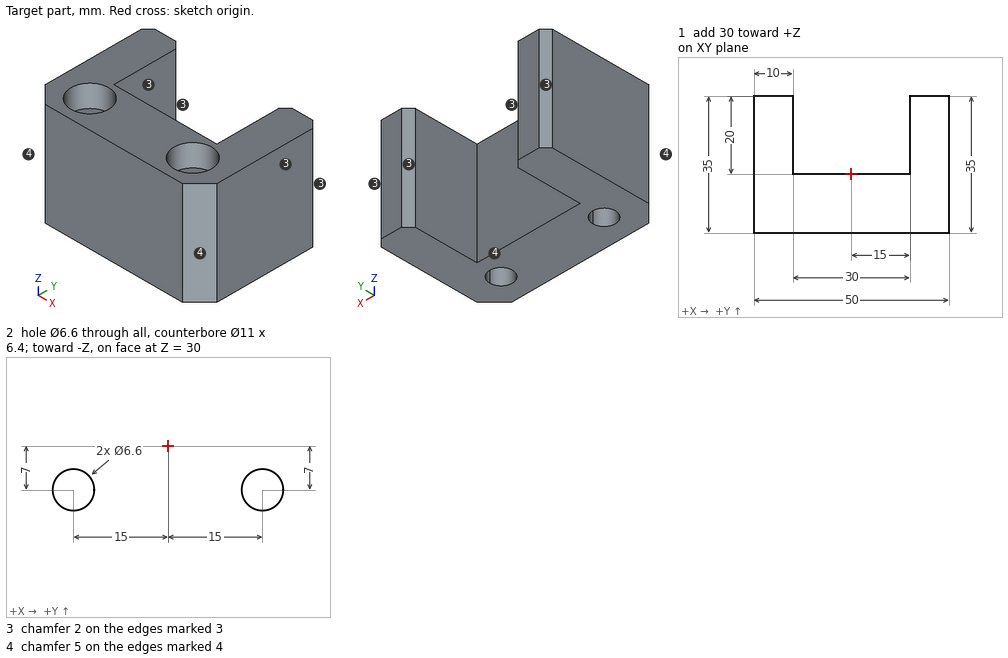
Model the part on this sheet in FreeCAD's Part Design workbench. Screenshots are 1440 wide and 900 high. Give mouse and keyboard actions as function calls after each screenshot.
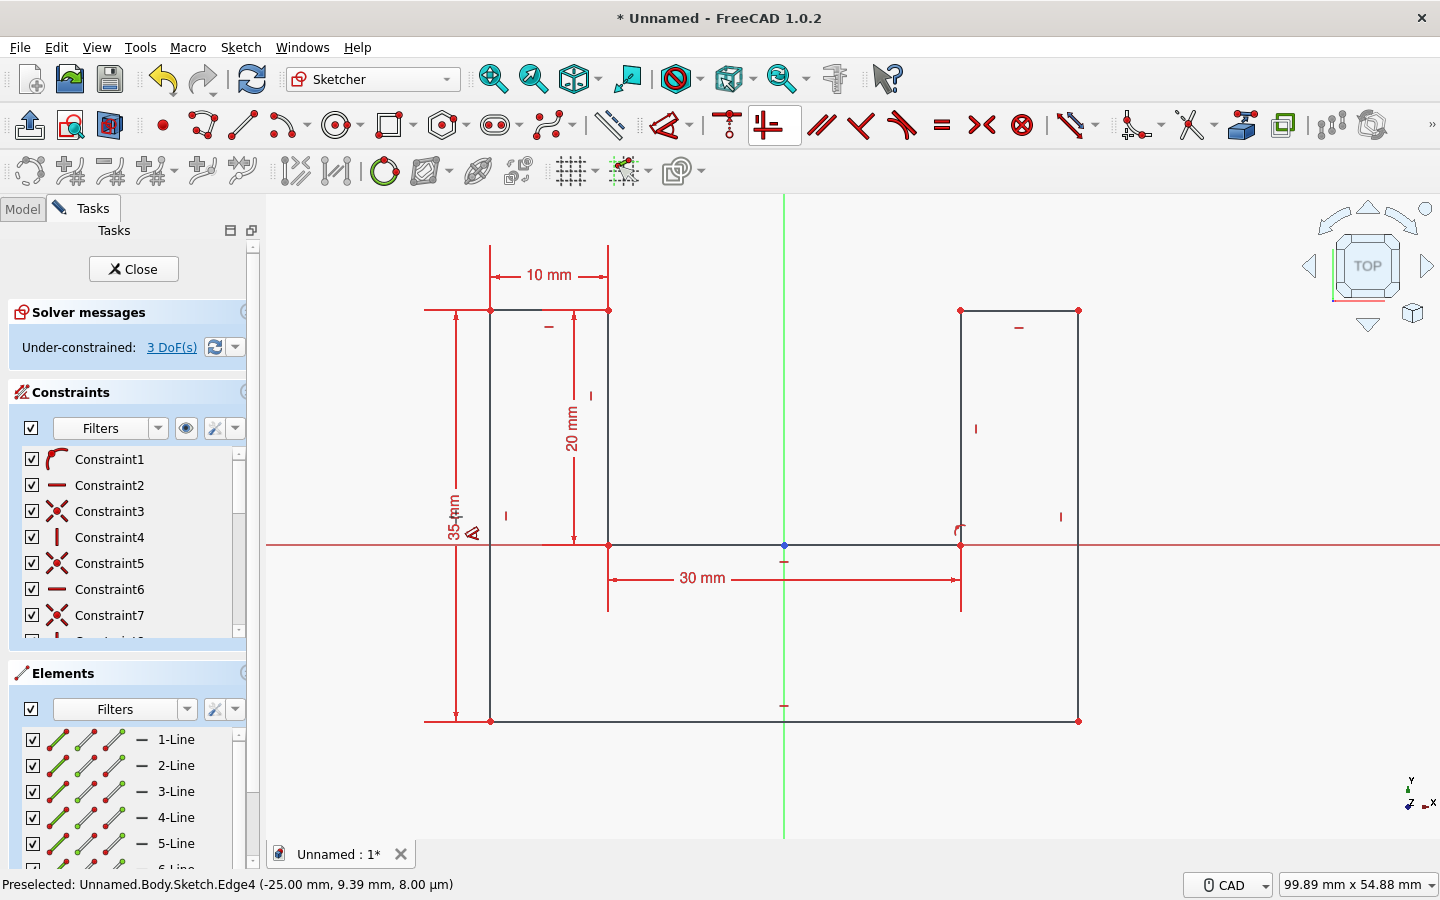
click(667, 722)
click(649, 756)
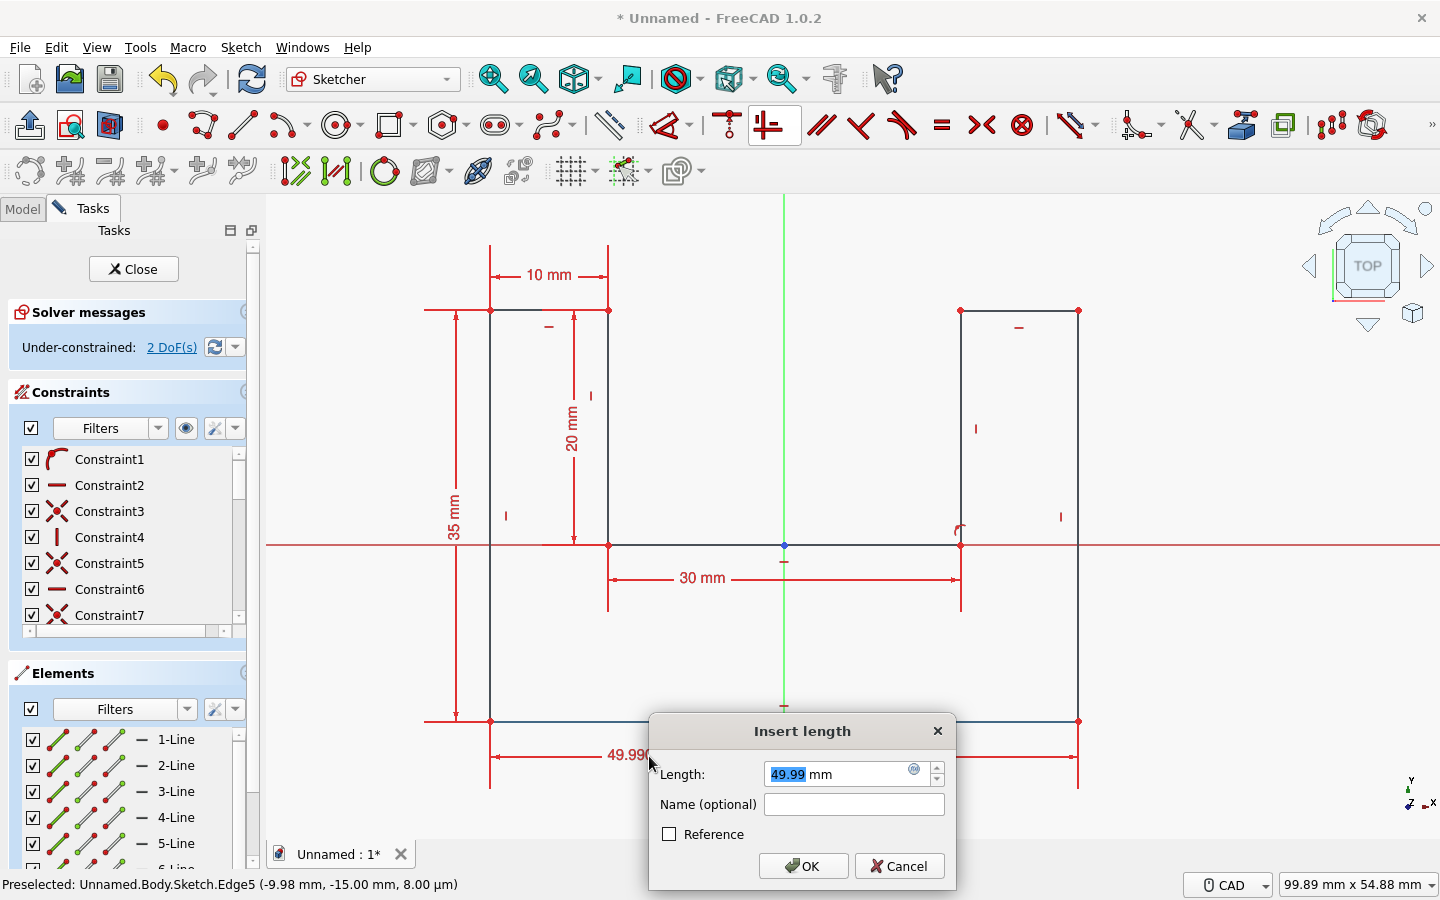
text(50)
key(Return)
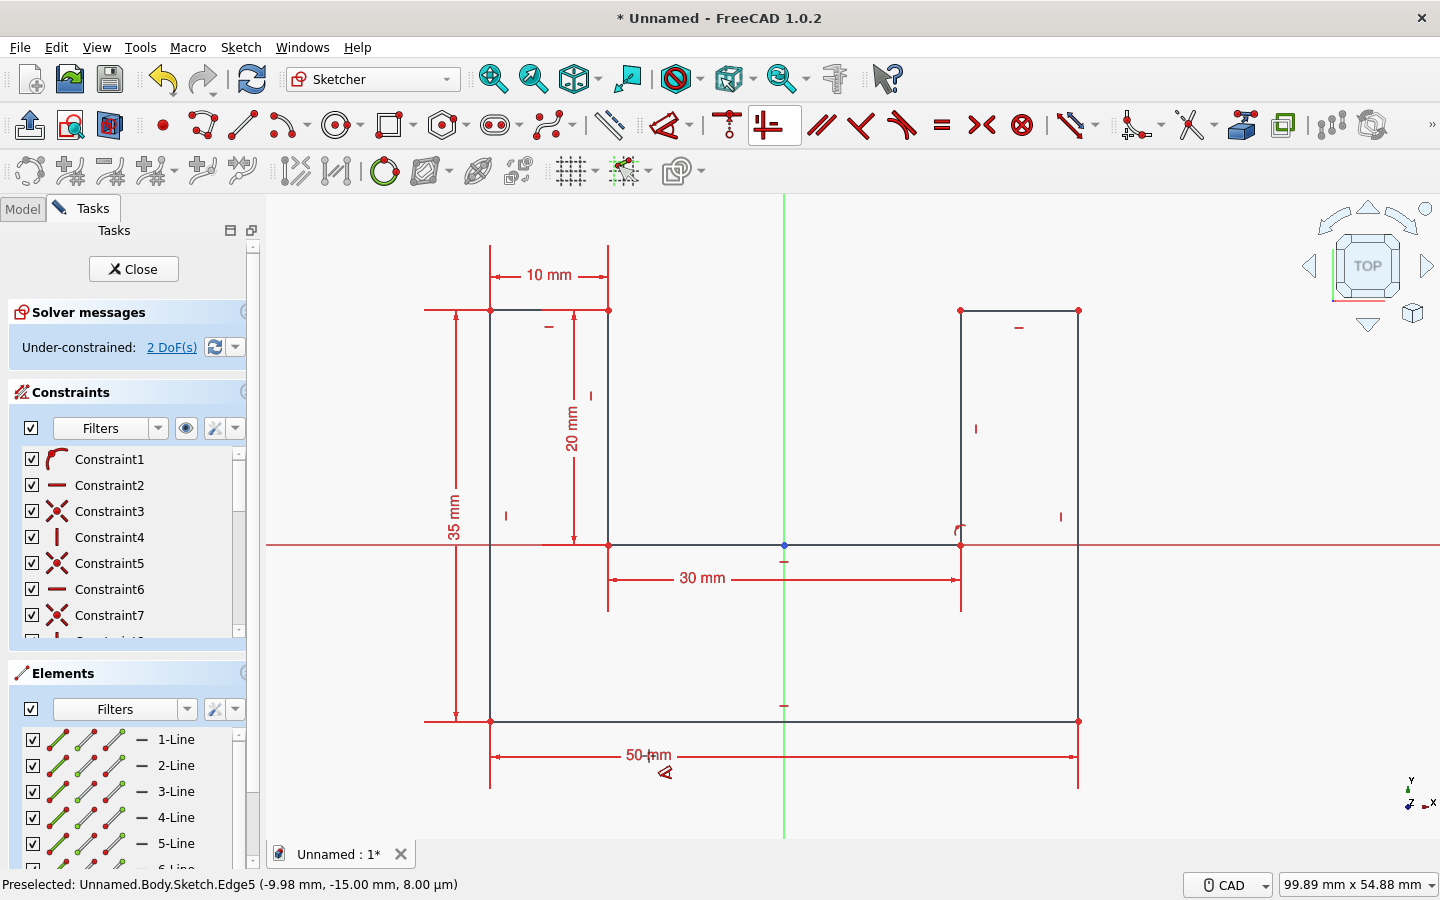
click(1078, 598)
click(1112, 516)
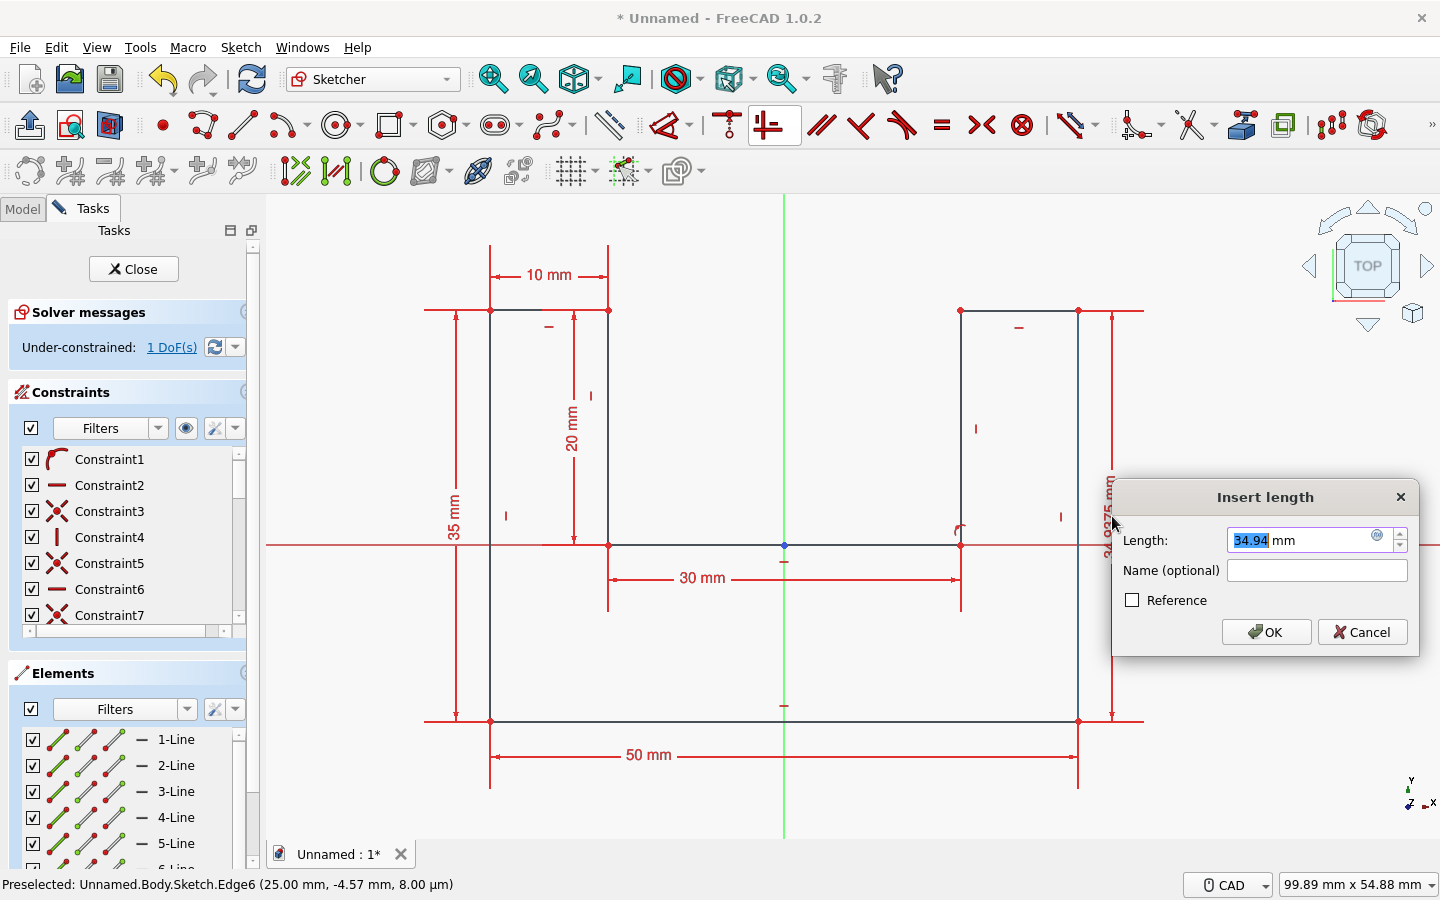
text(35)
key(Return)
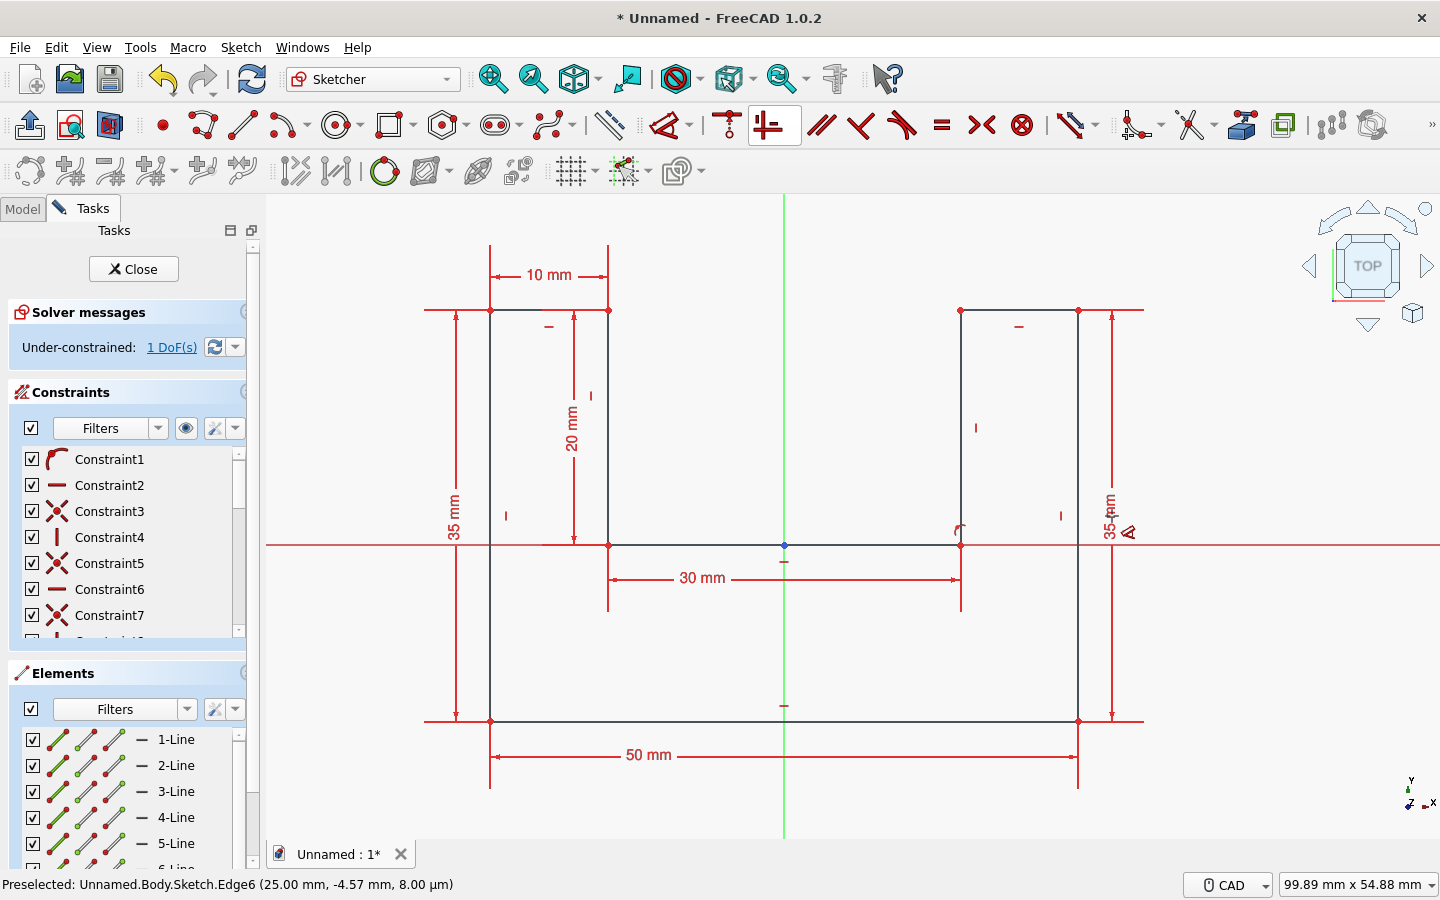
click(961, 545)
click(872, 579)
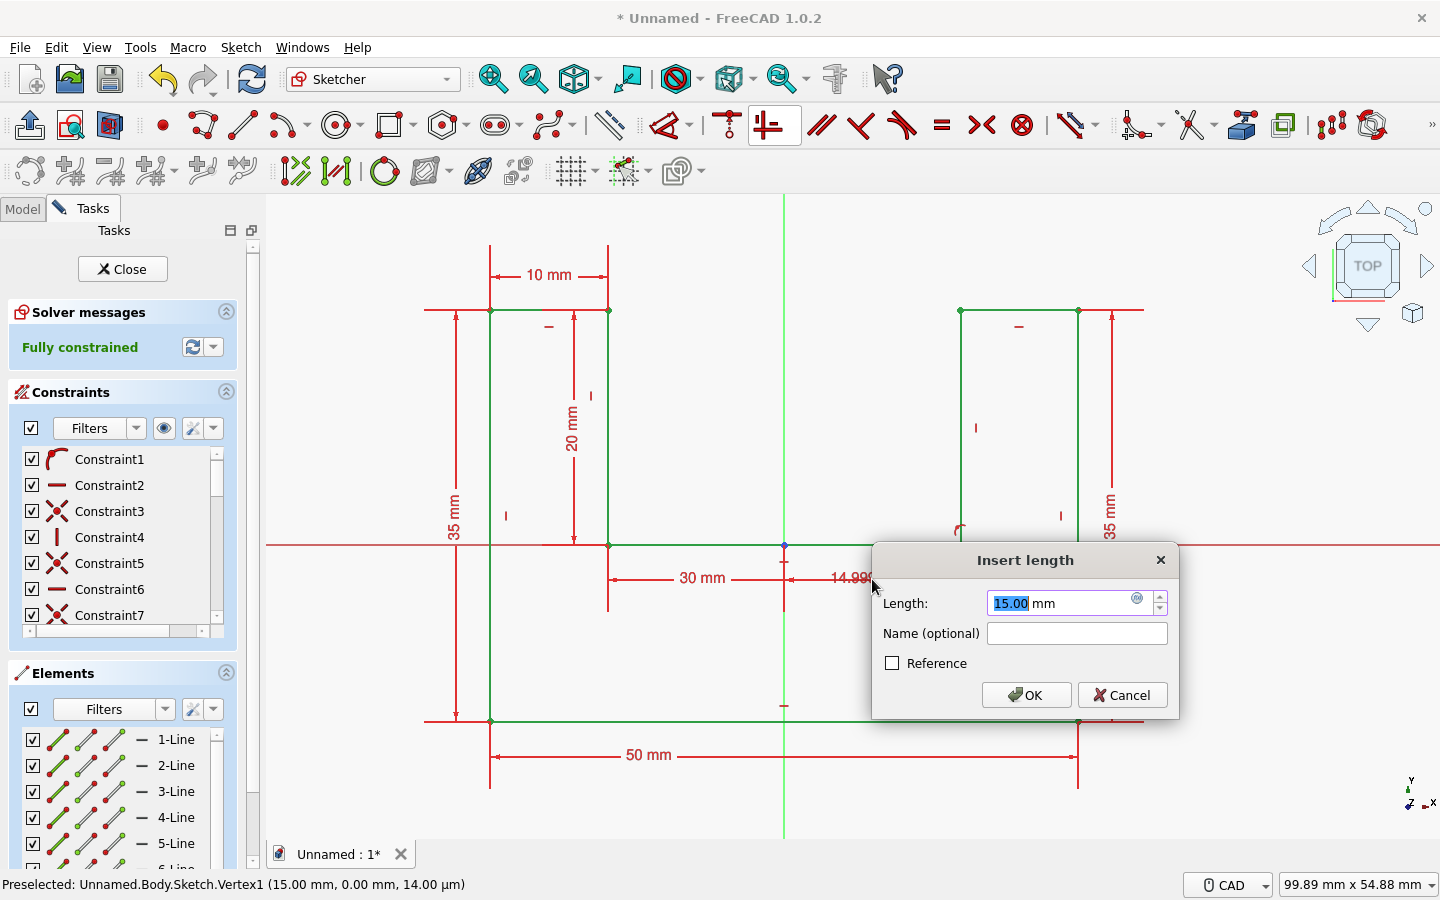
text(15)
key(Return)
key(Escape)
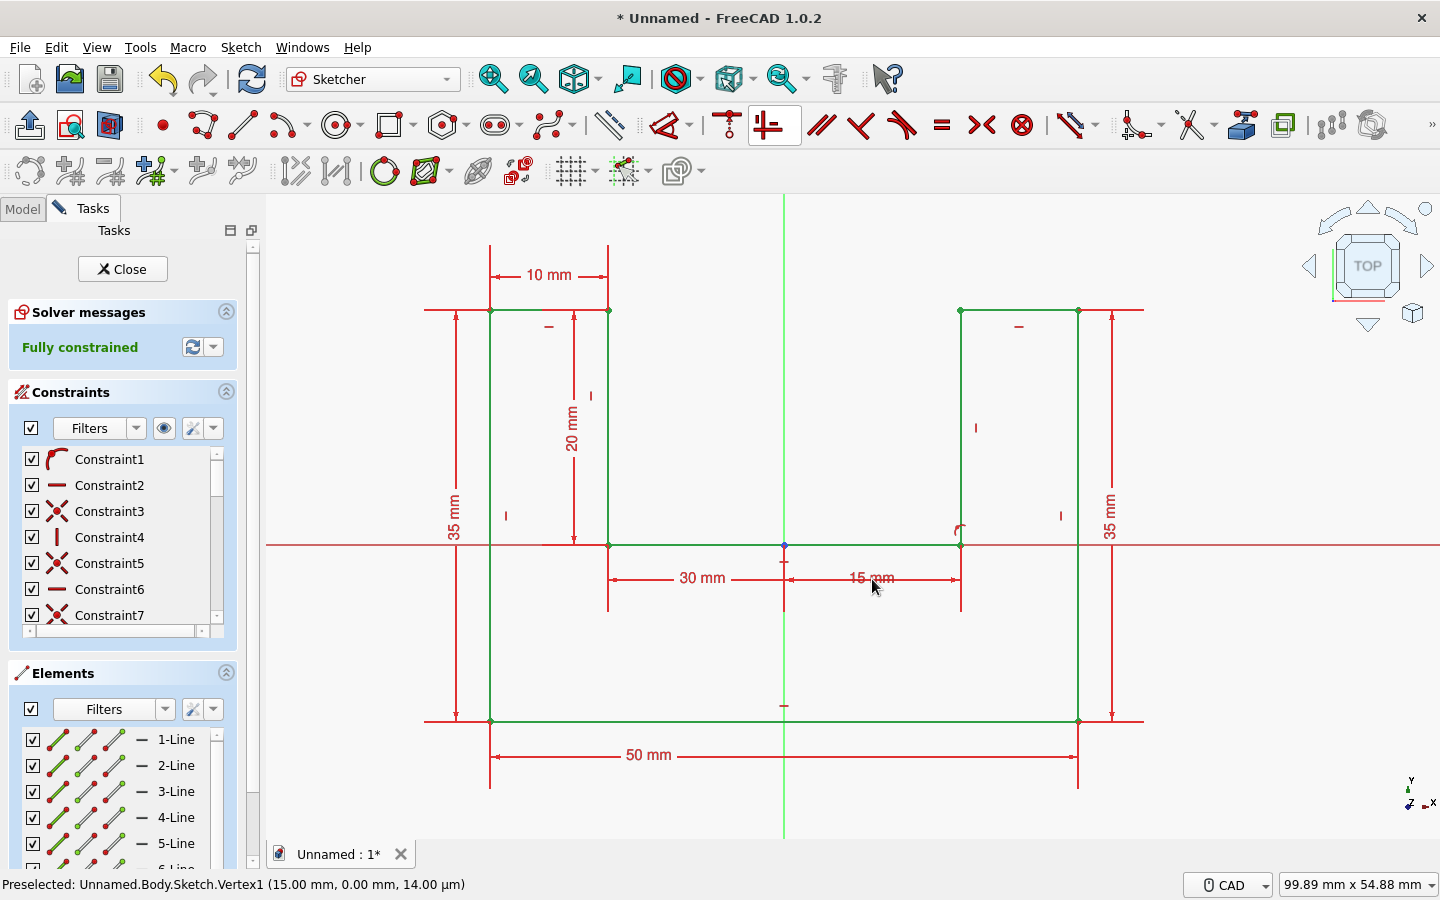
click(123, 269)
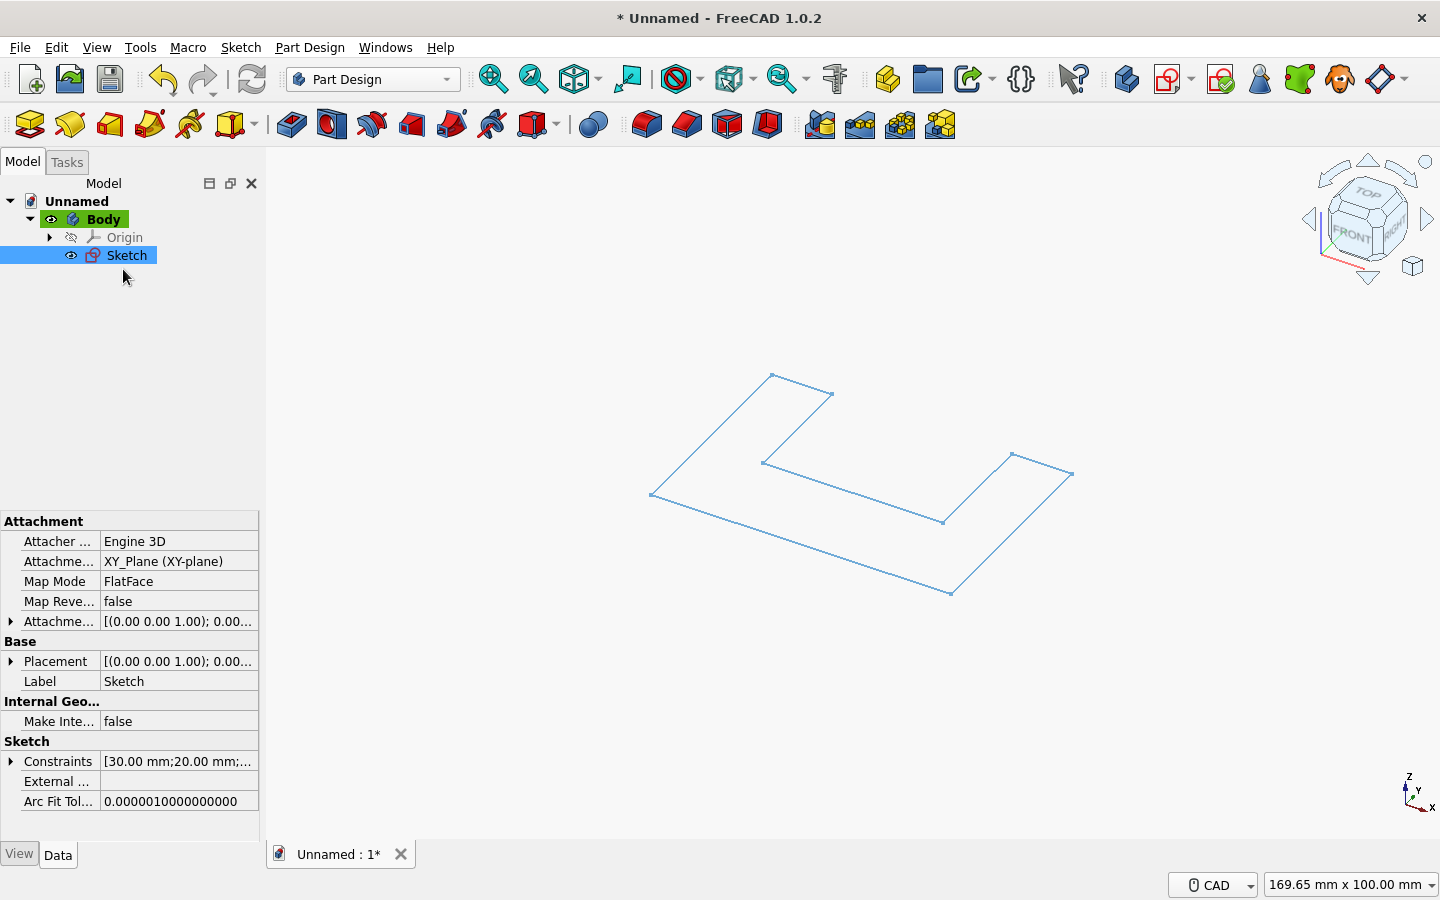
click(30, 124)